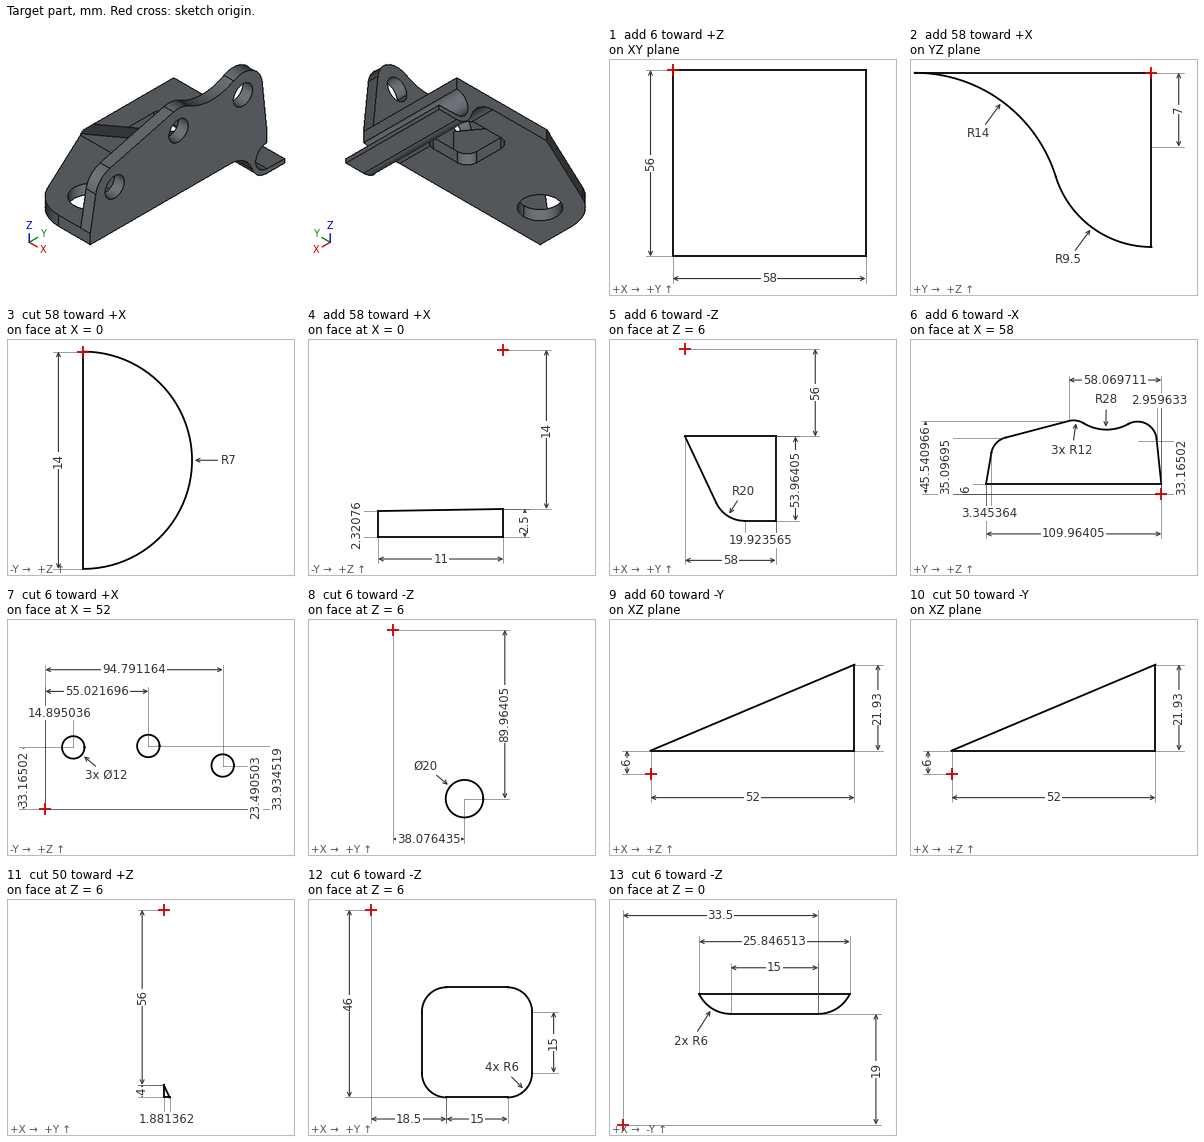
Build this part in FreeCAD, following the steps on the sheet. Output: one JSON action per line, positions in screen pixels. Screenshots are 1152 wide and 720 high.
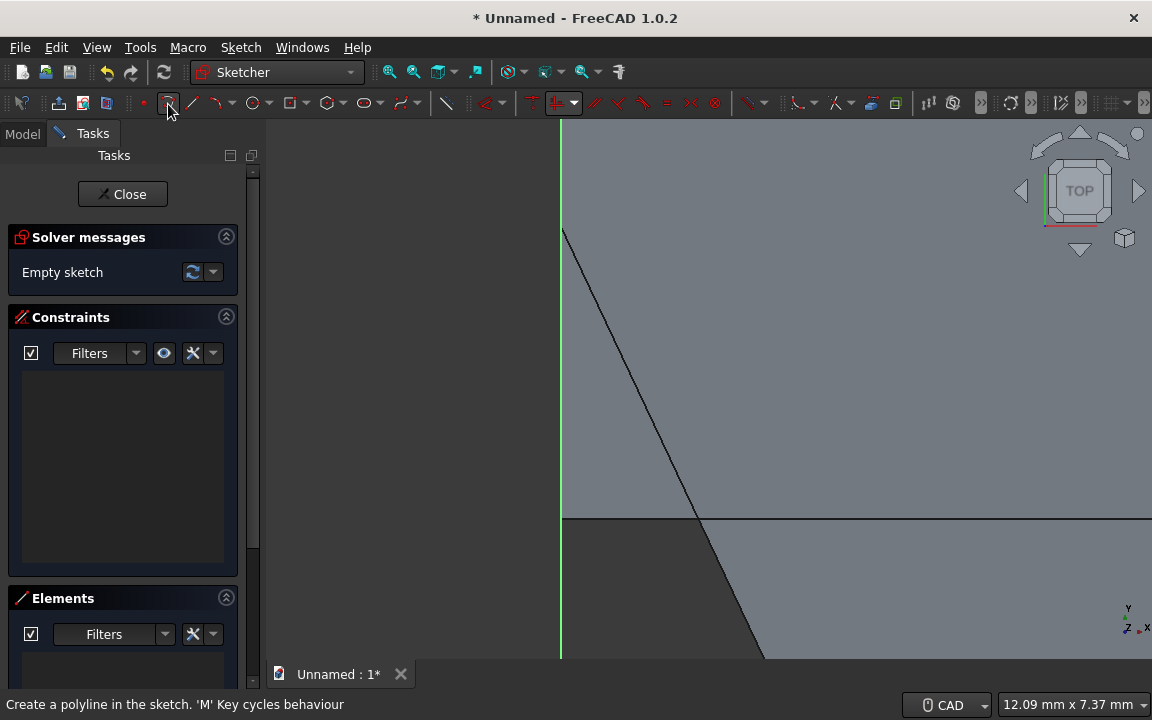
{"action": "left_click", "coordinate": [561, 226]}
{"action": "left_click", "coordinate": [699, 519]}
{"action": "left_click", "coordinate": [570, 519]}
{"action": "left_click", "coordinate": [561, 227]}
{"action": "key", "text": "Escape"}
{"action": "key", "text": "Escape"}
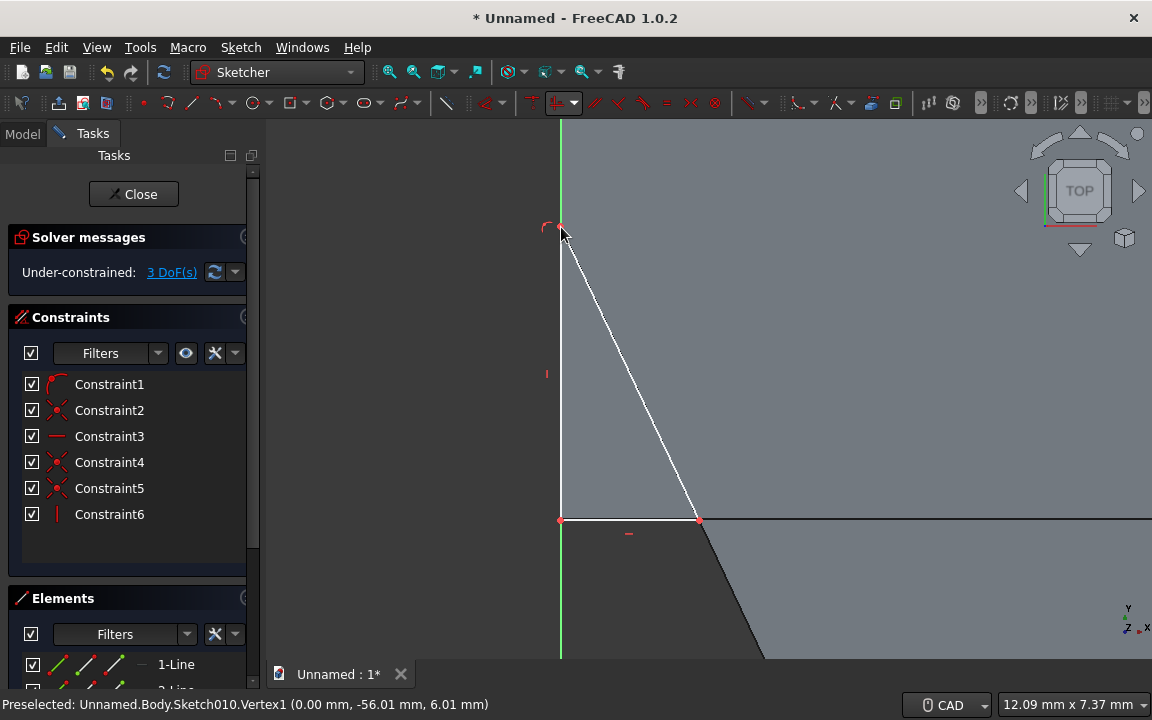
{"action": "left_click", "coordinate": [486, 104]}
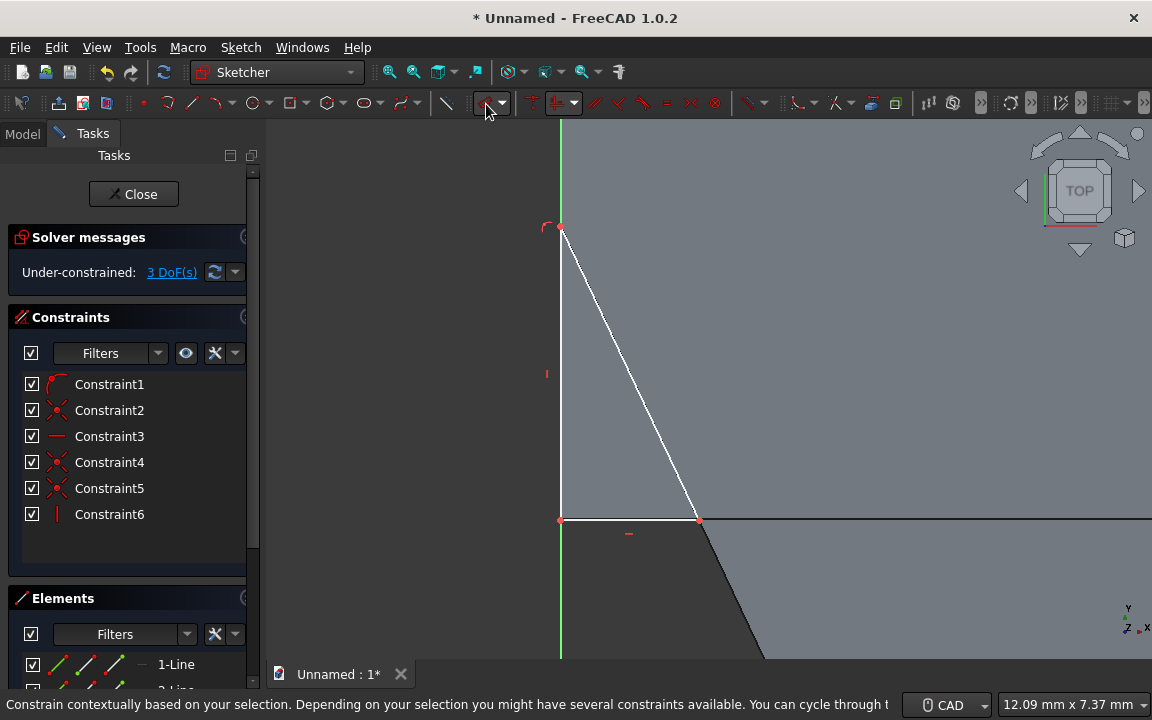
{"action": "left_click", "coordinate": [561, 432]}
{"action": "left_click", "coordinate": [527, 374]}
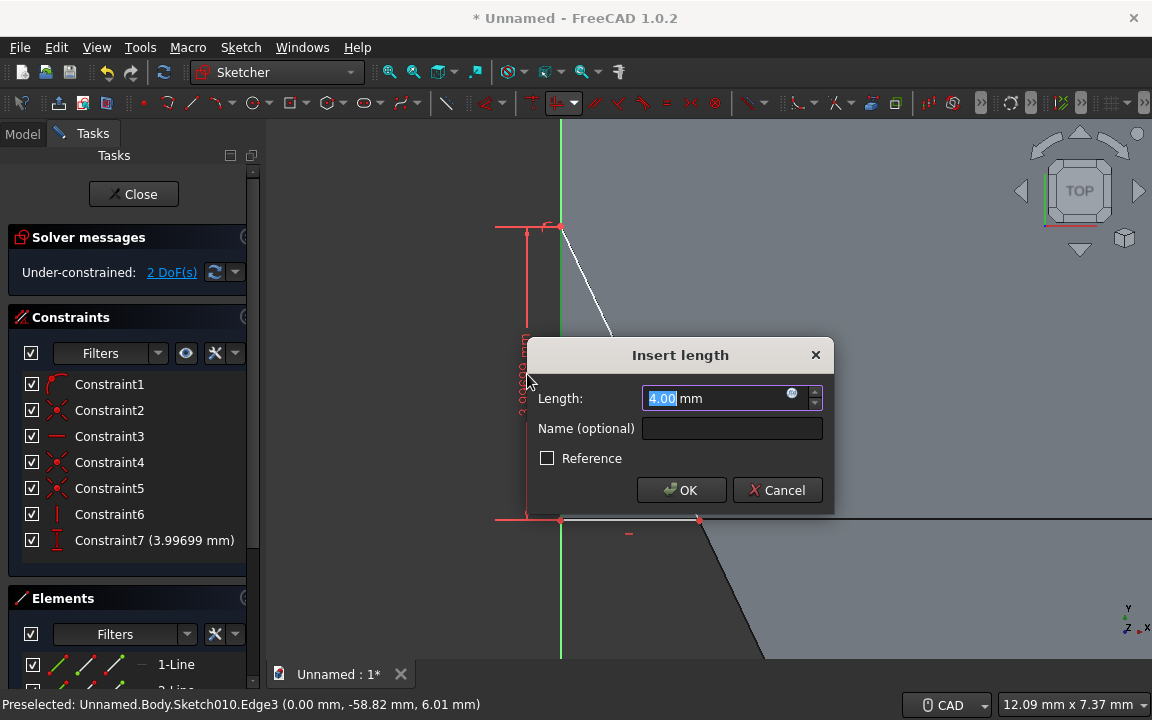
{"action": "type", "text": "4"}
{"action": "key", "text": "Return"}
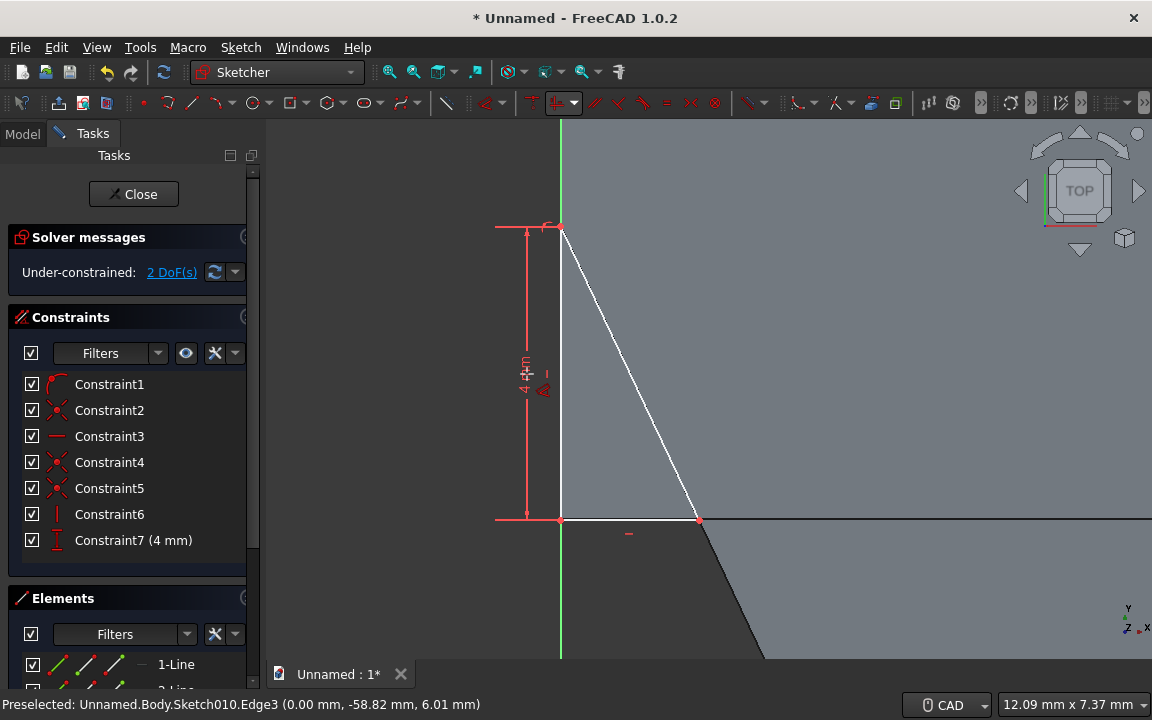
{"action": "left_click", "coordinate": [561, 227]}
{"action": "left_click", "coordinate": [527, 187]}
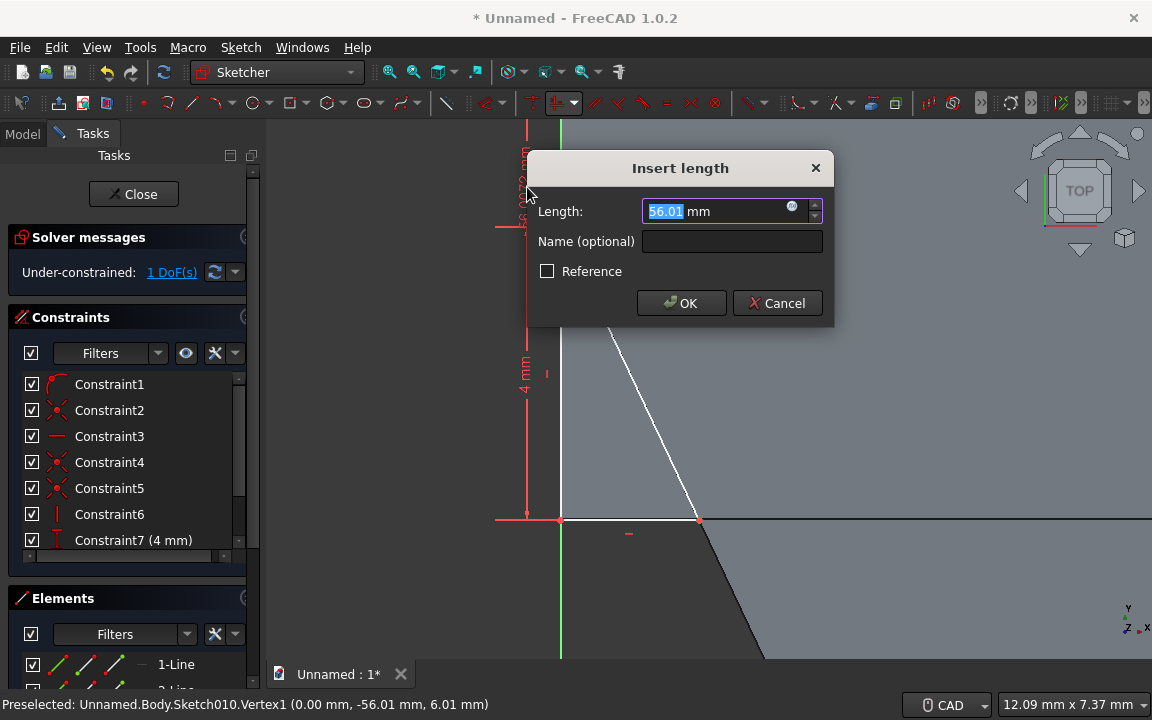
{"action": "type", "text": "56"}
{"action": "key", "text": "Return"}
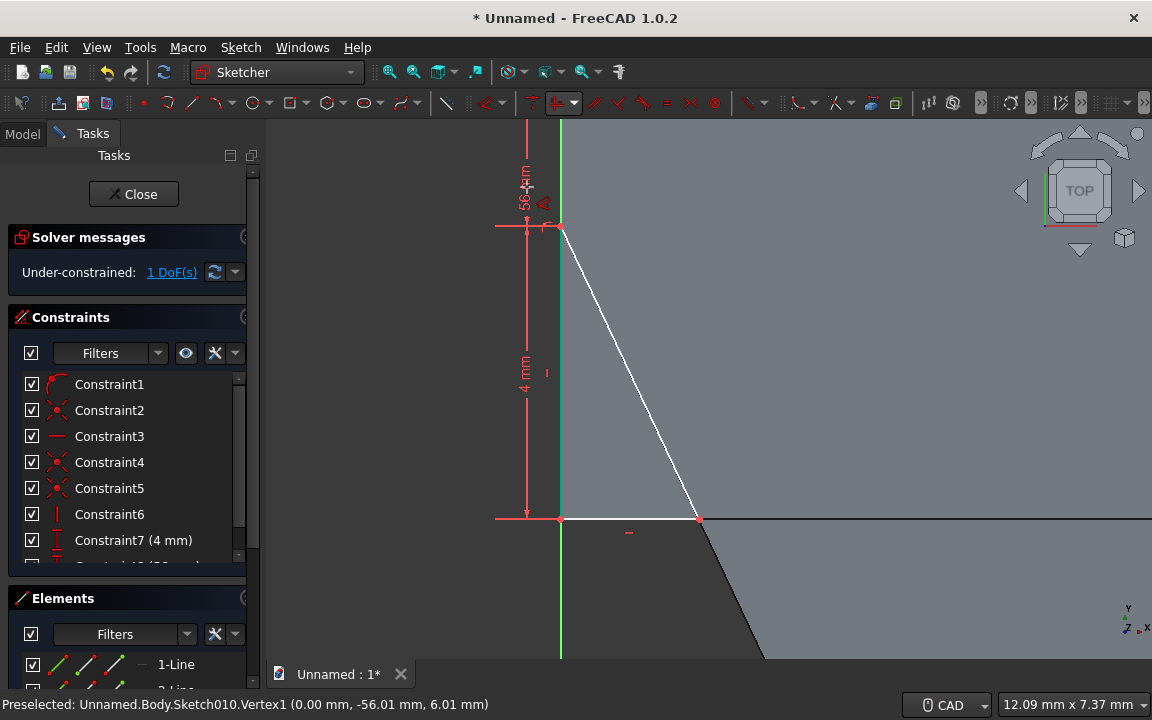
{"action": "left_click", "coordinate": [658, 519]}
{"action": "left_click", "coordinate": [630, 553]}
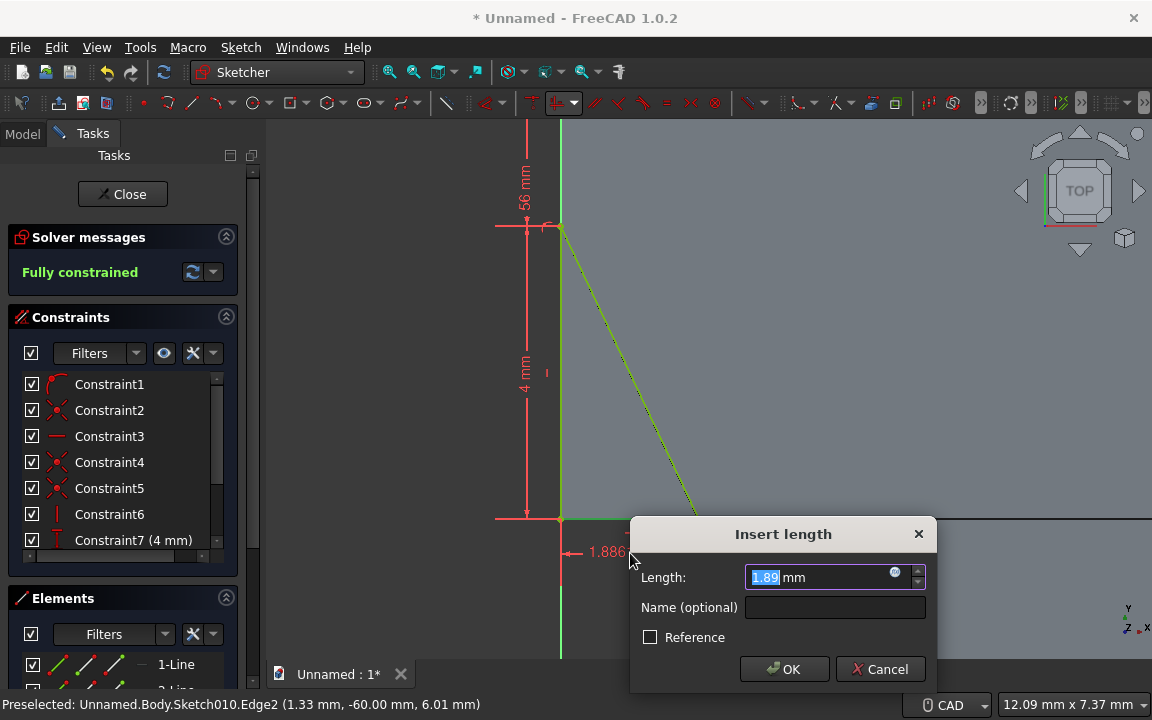
{"action": "type", "text": "1.881362"}
{"action": "key", "text": "Return"}
{"action": "key", "text": "Escape"}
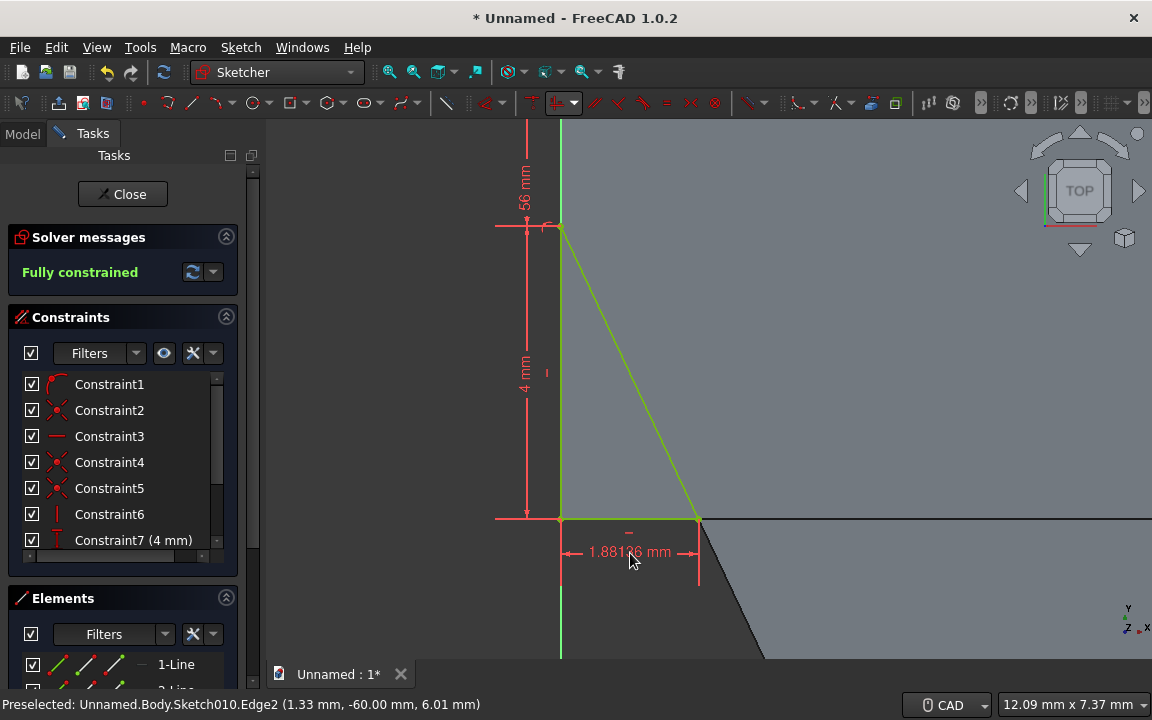
{"action": "left_click", "coordinate": [123, 194]}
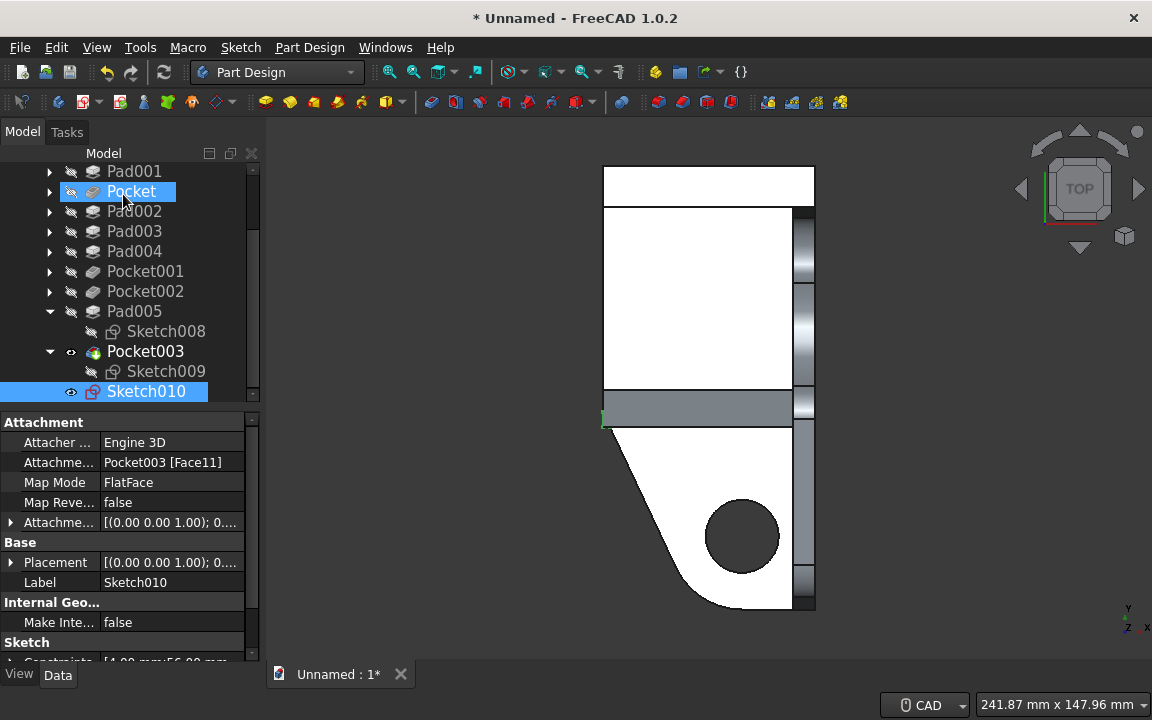
{"action": "left_click", "coordinate": [432, 102]}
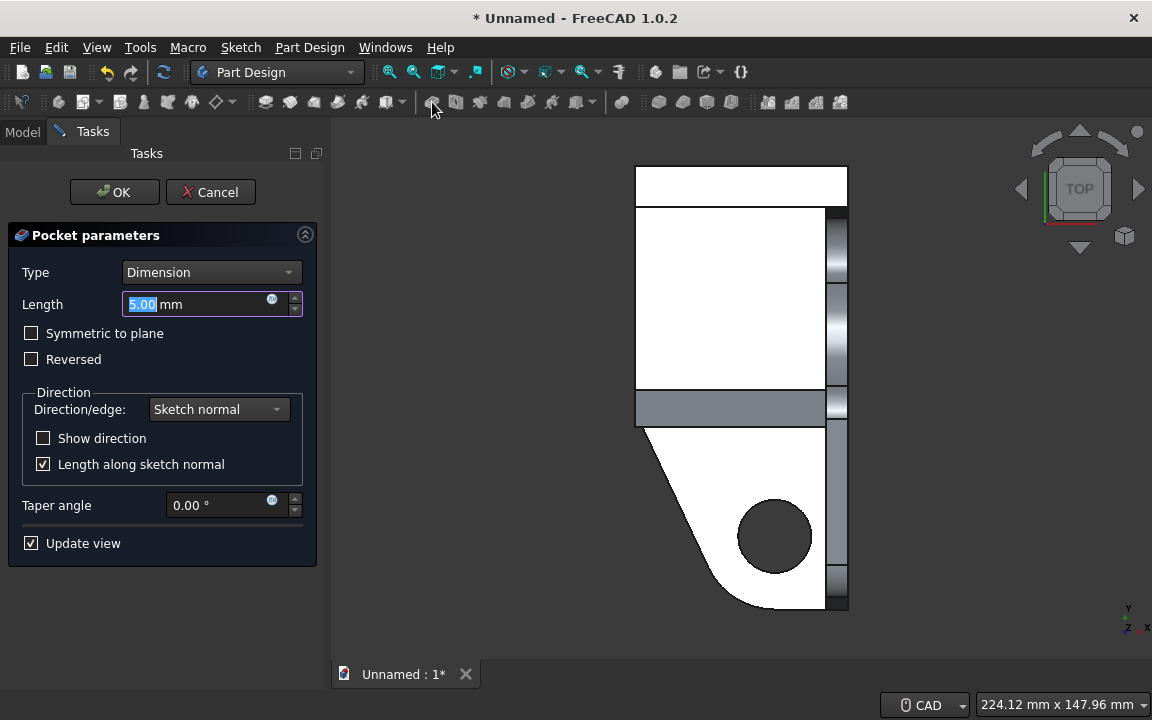
{"action": "type", "text": "50"}
{"action": "key", "text": "Tab"}